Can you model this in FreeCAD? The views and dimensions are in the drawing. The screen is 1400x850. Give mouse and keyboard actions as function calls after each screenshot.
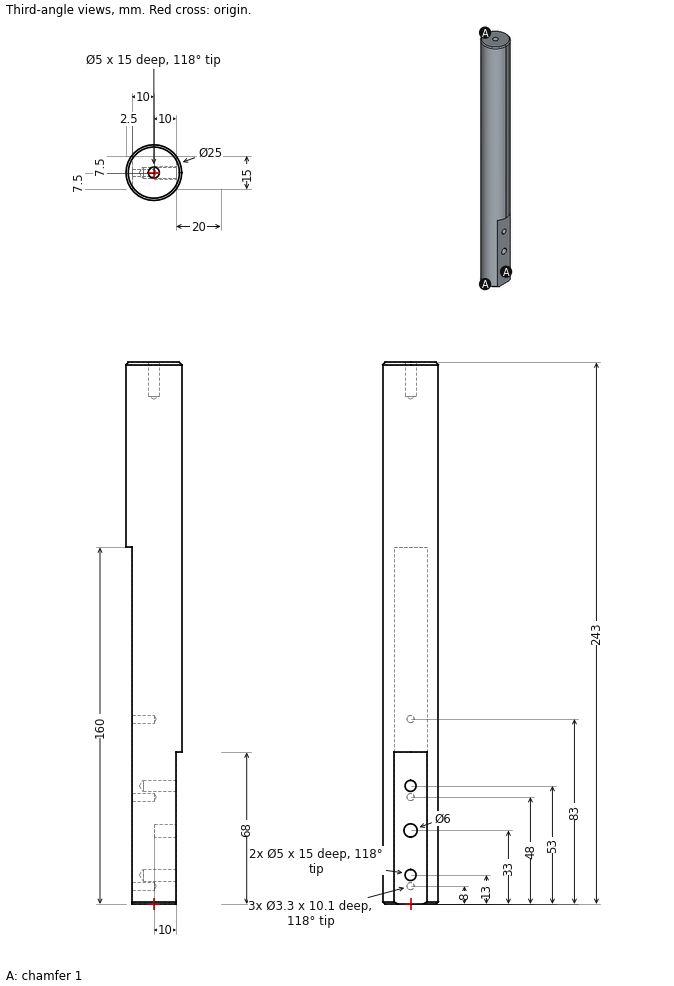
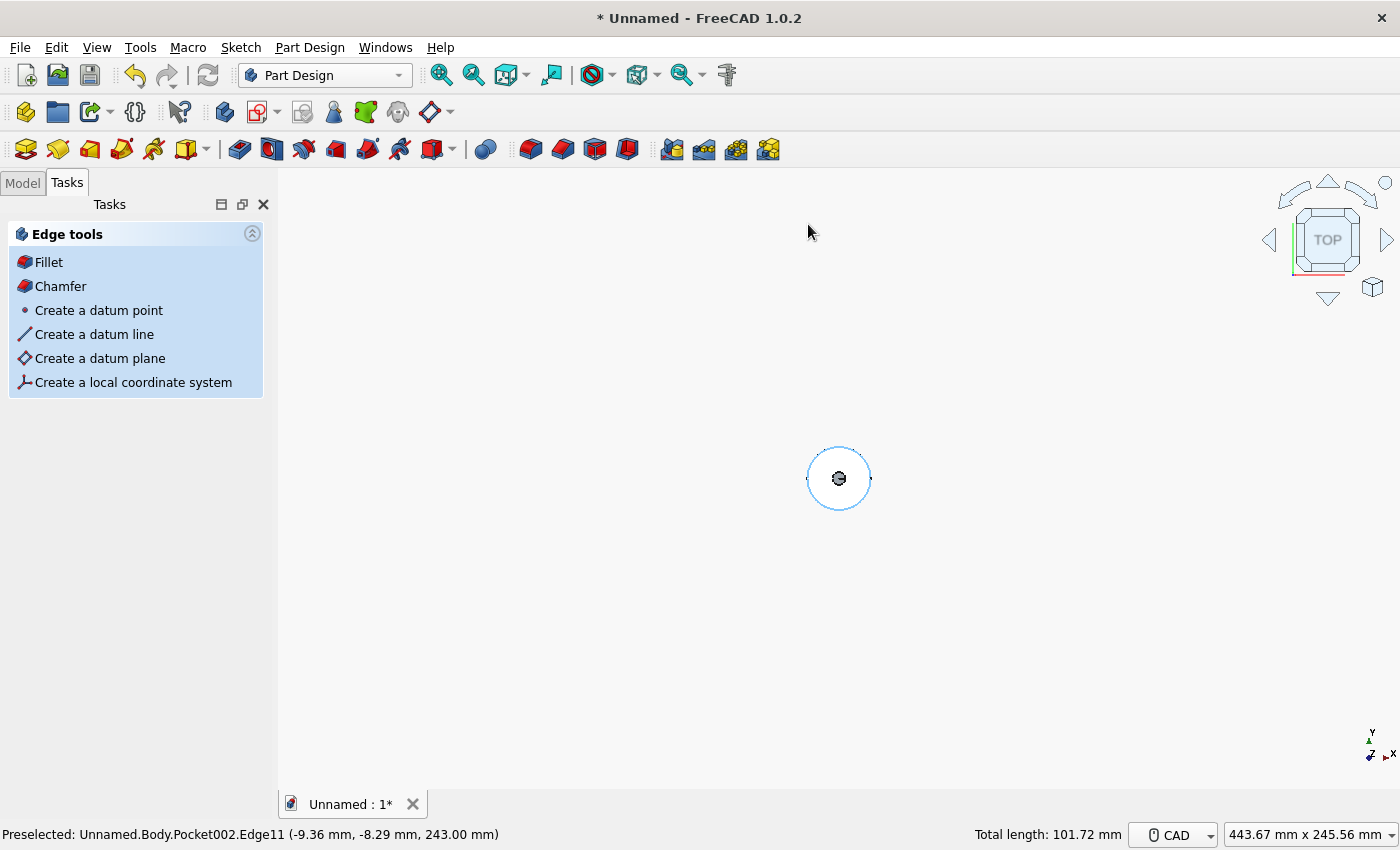
key(v)
key(f)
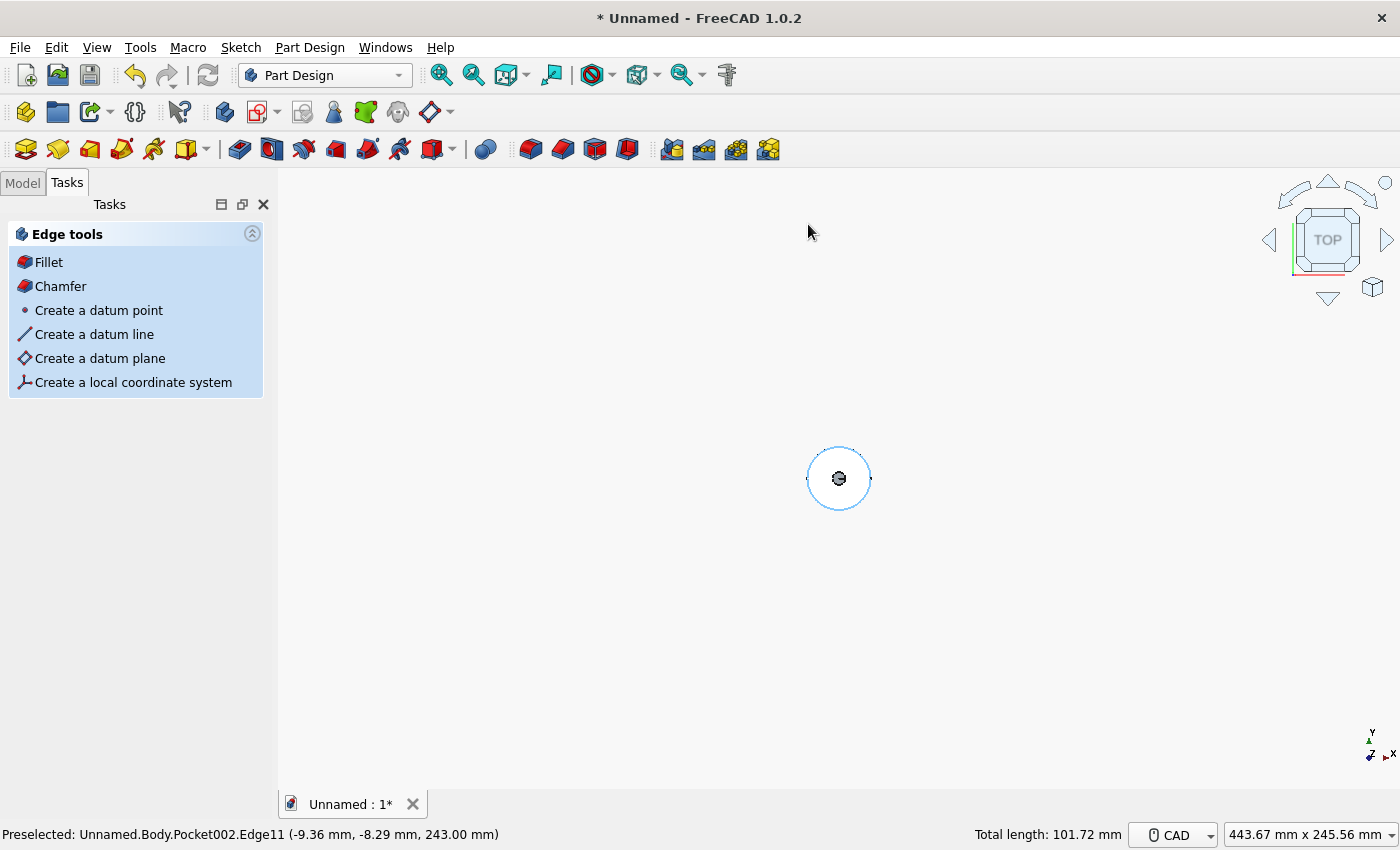
key(0)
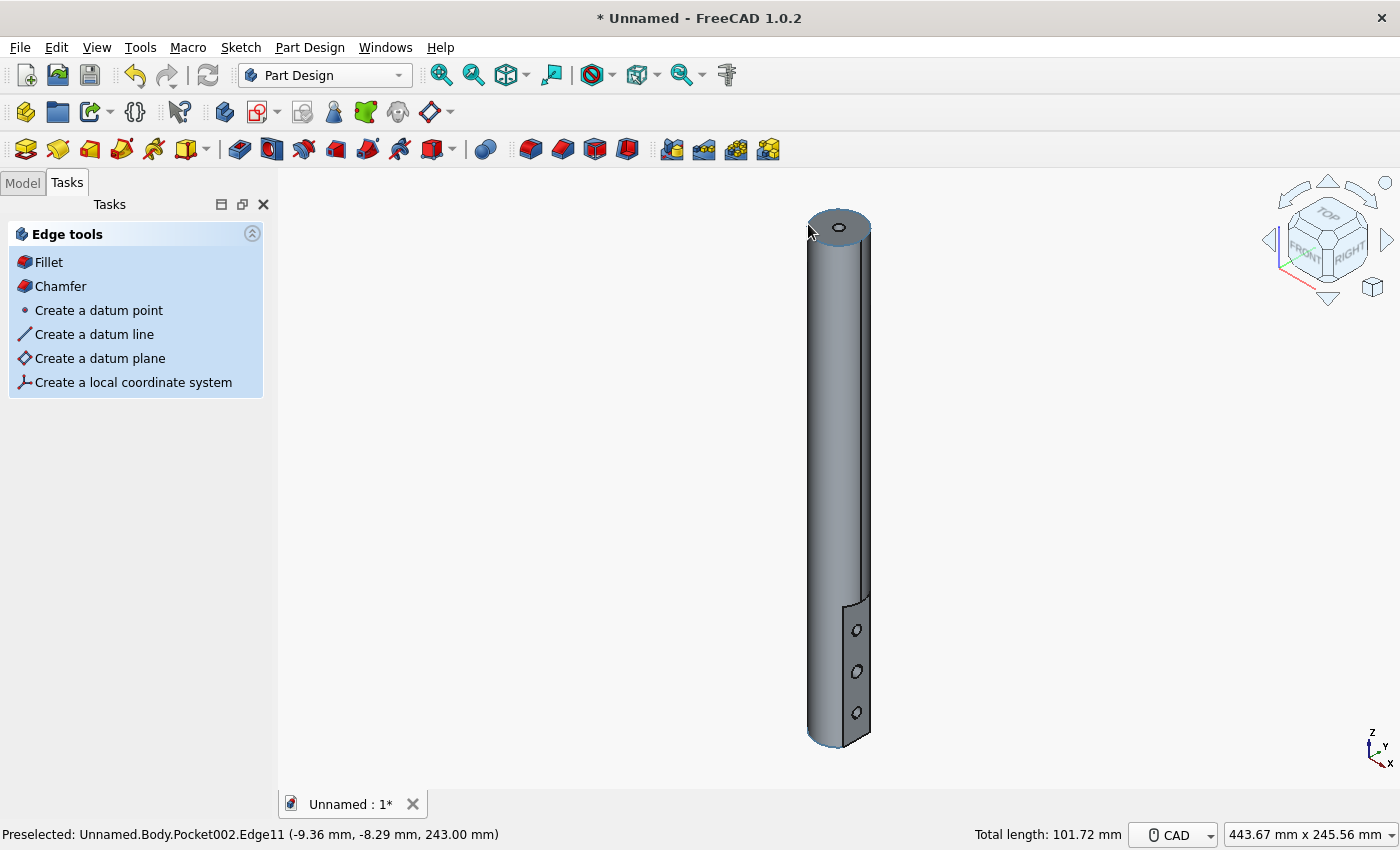
key(1)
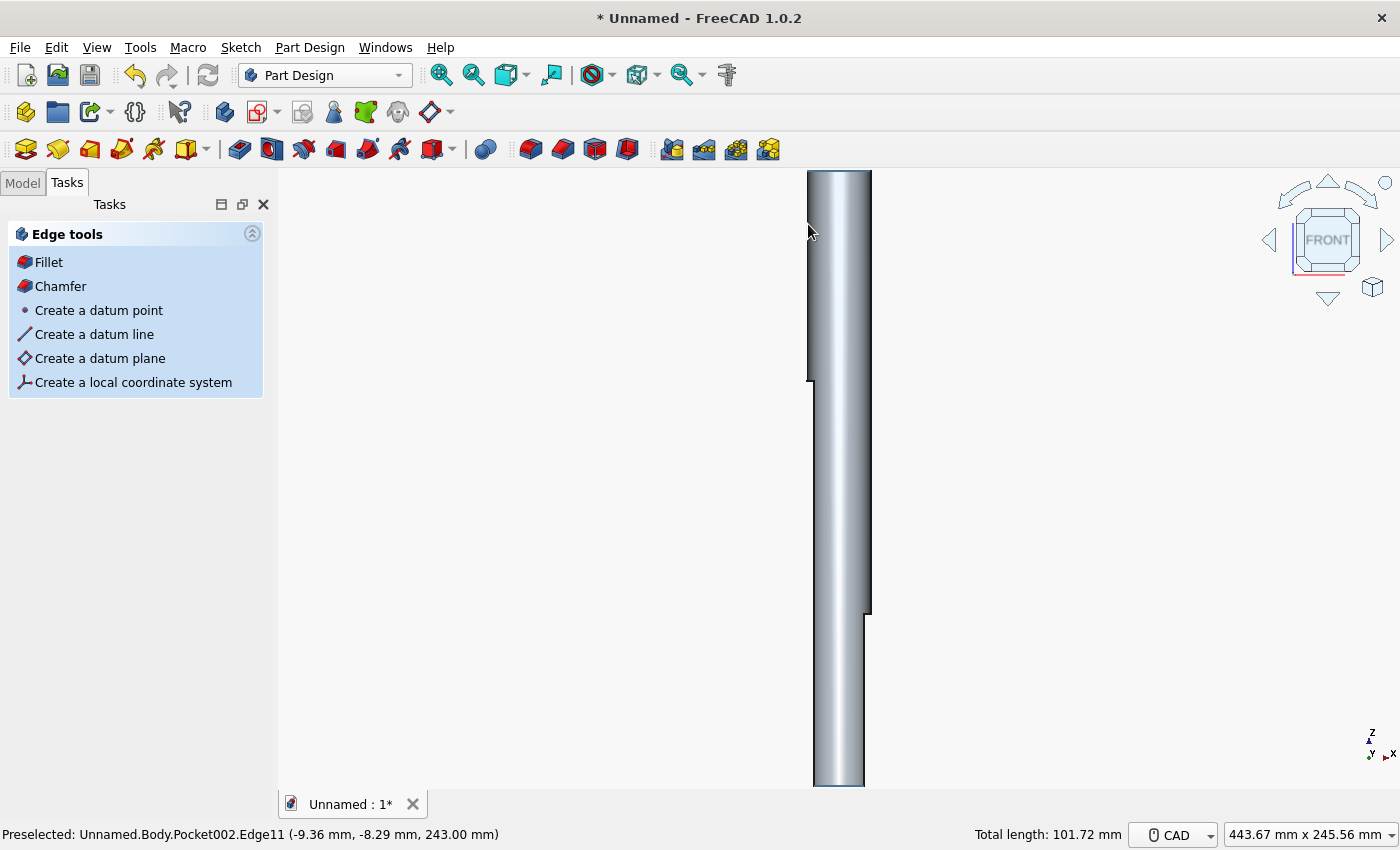
key(3)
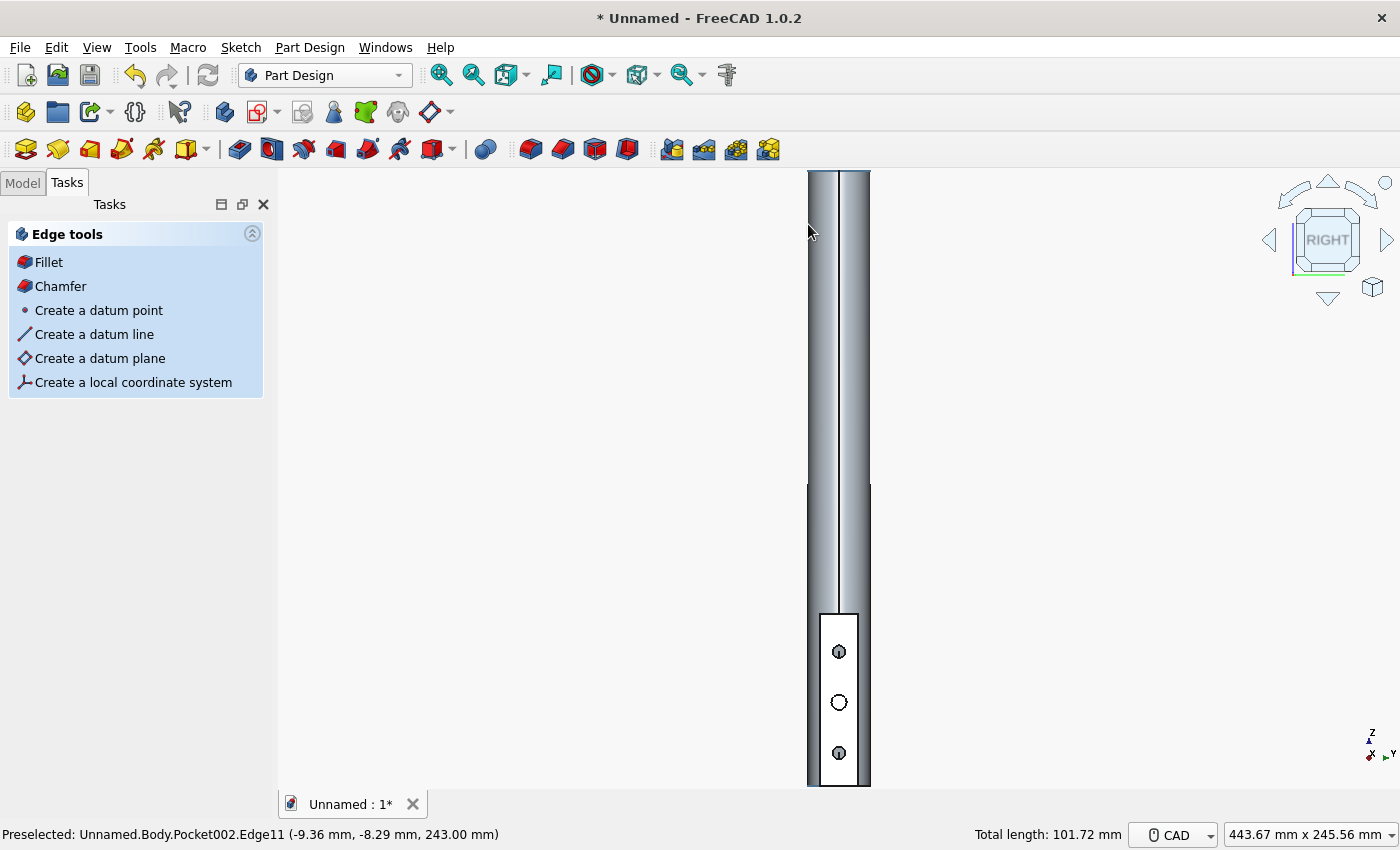
key(5)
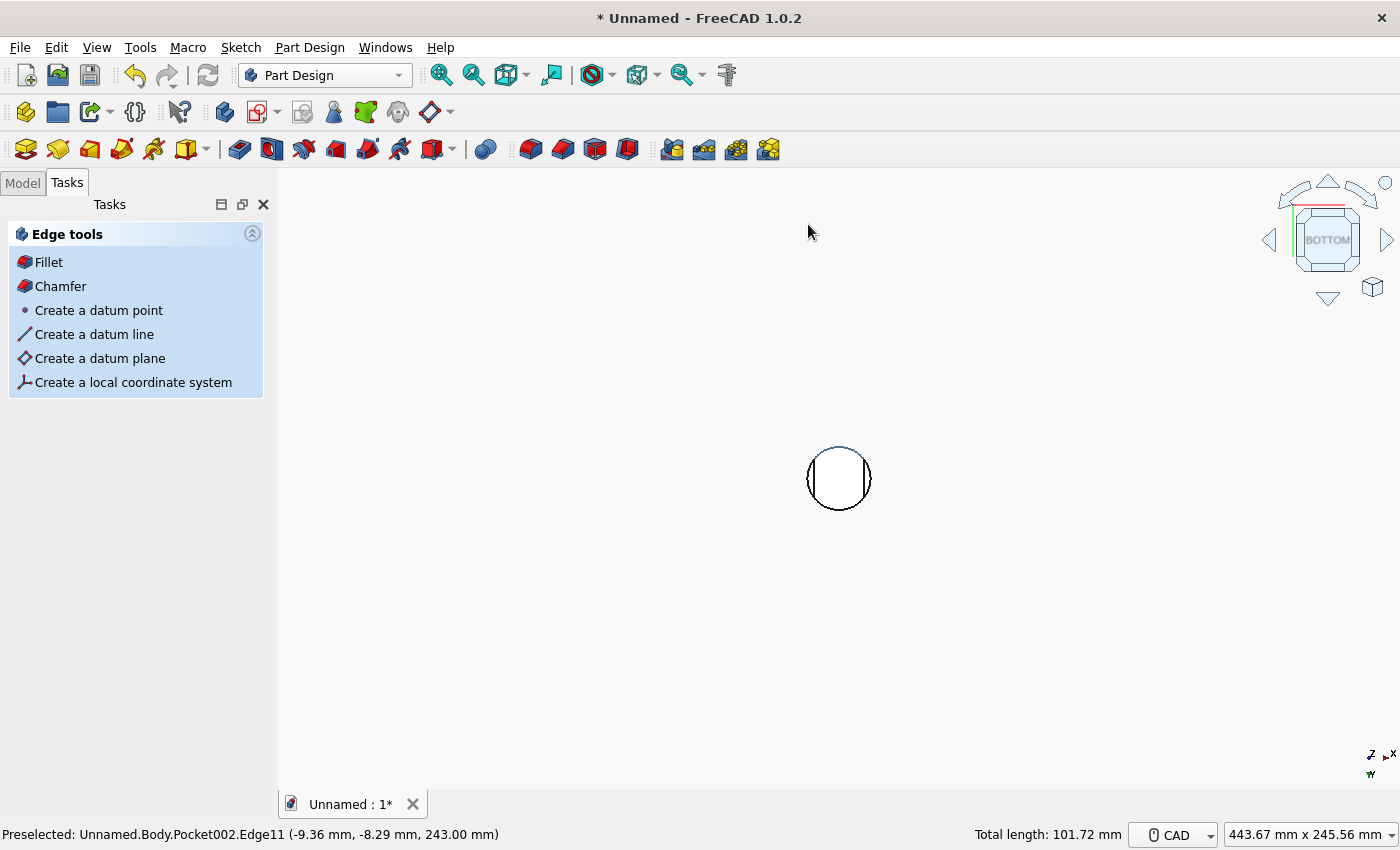
key(v)
key(f)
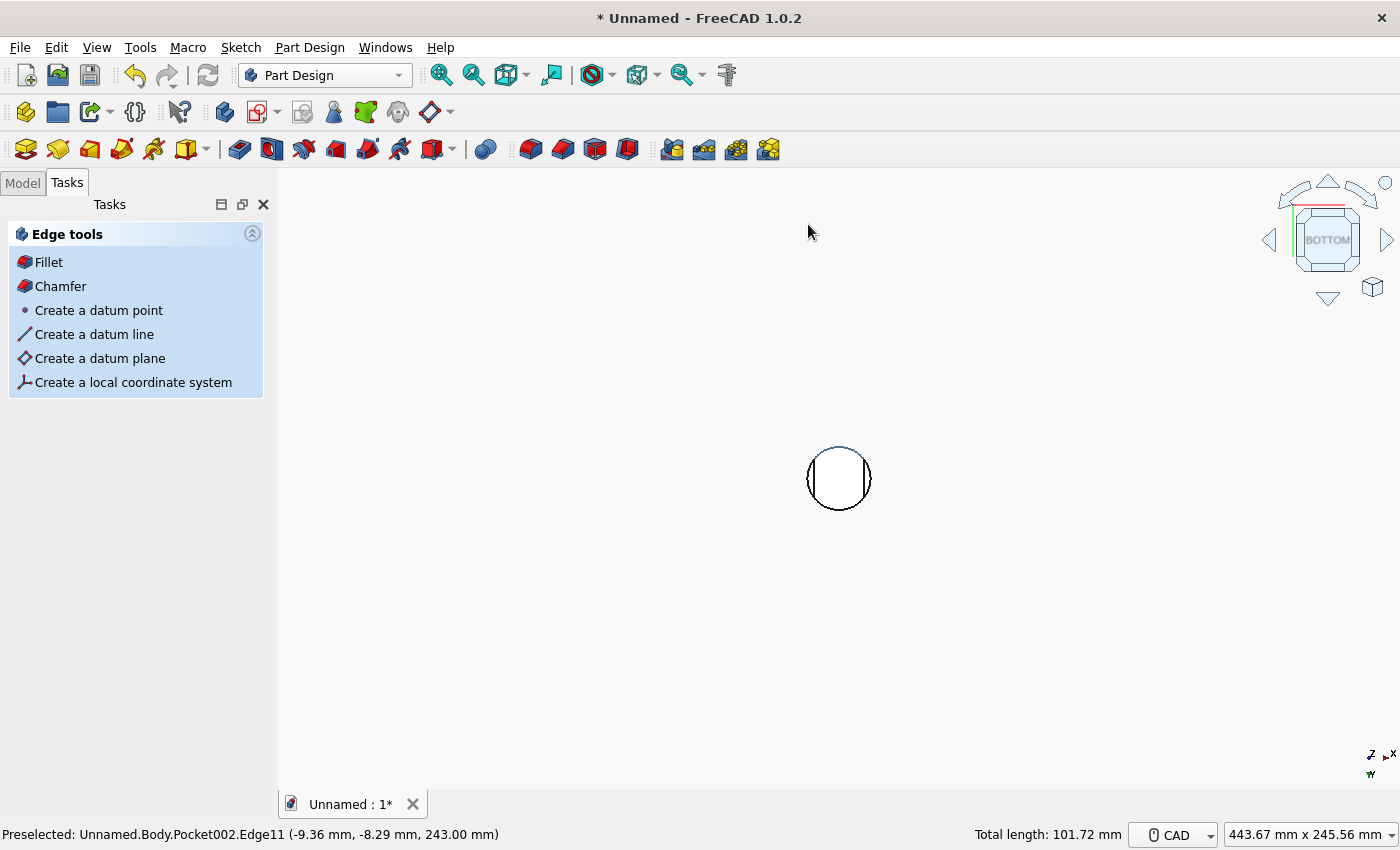
click(839, 509, ctrl)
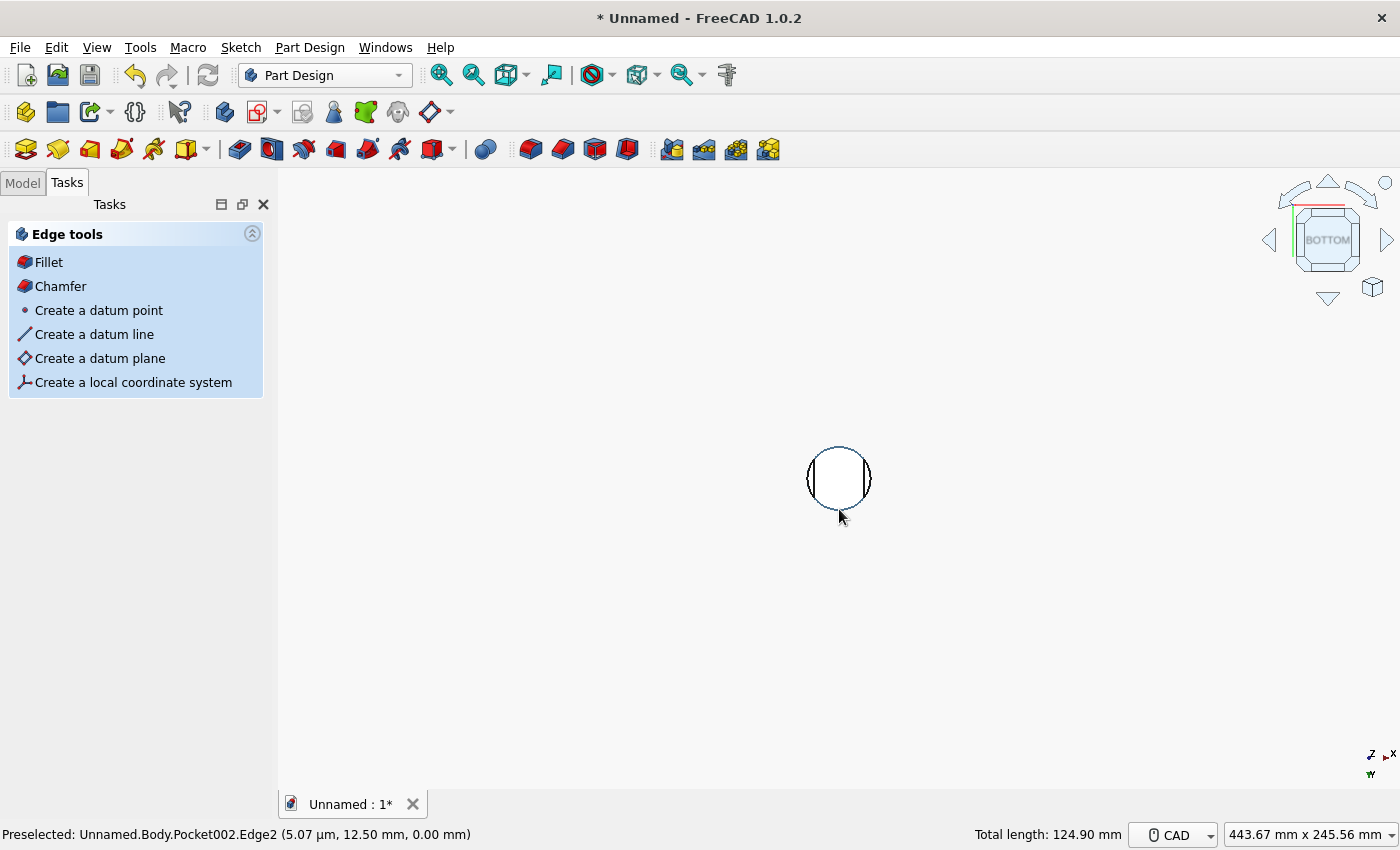
click(564, 150)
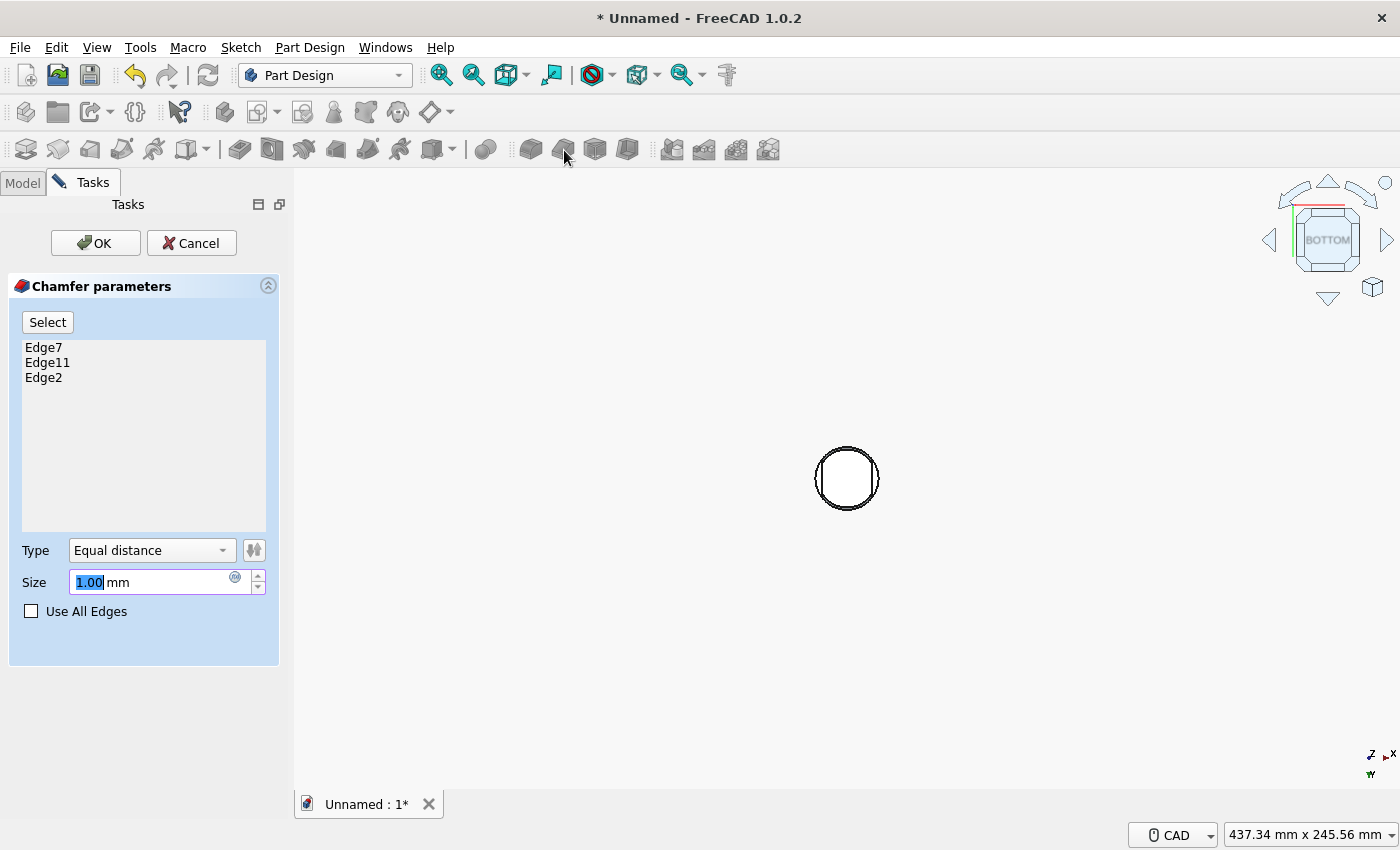
text(1)
key(Tab)